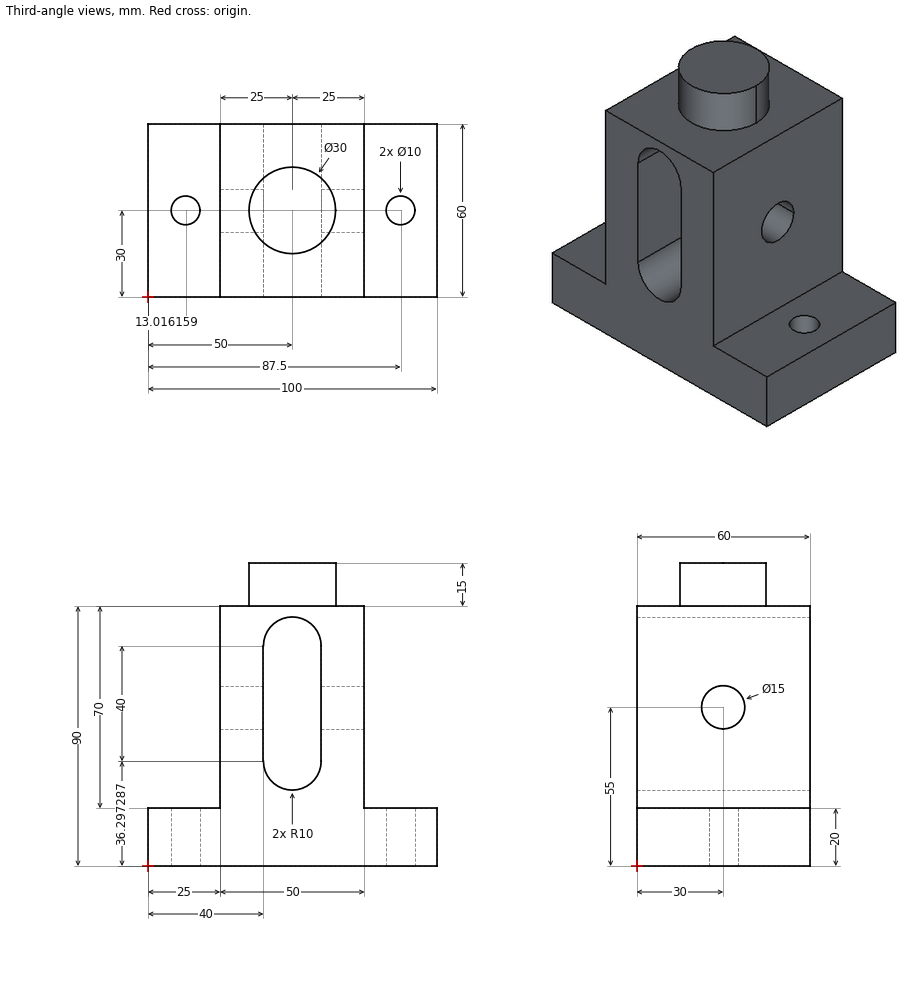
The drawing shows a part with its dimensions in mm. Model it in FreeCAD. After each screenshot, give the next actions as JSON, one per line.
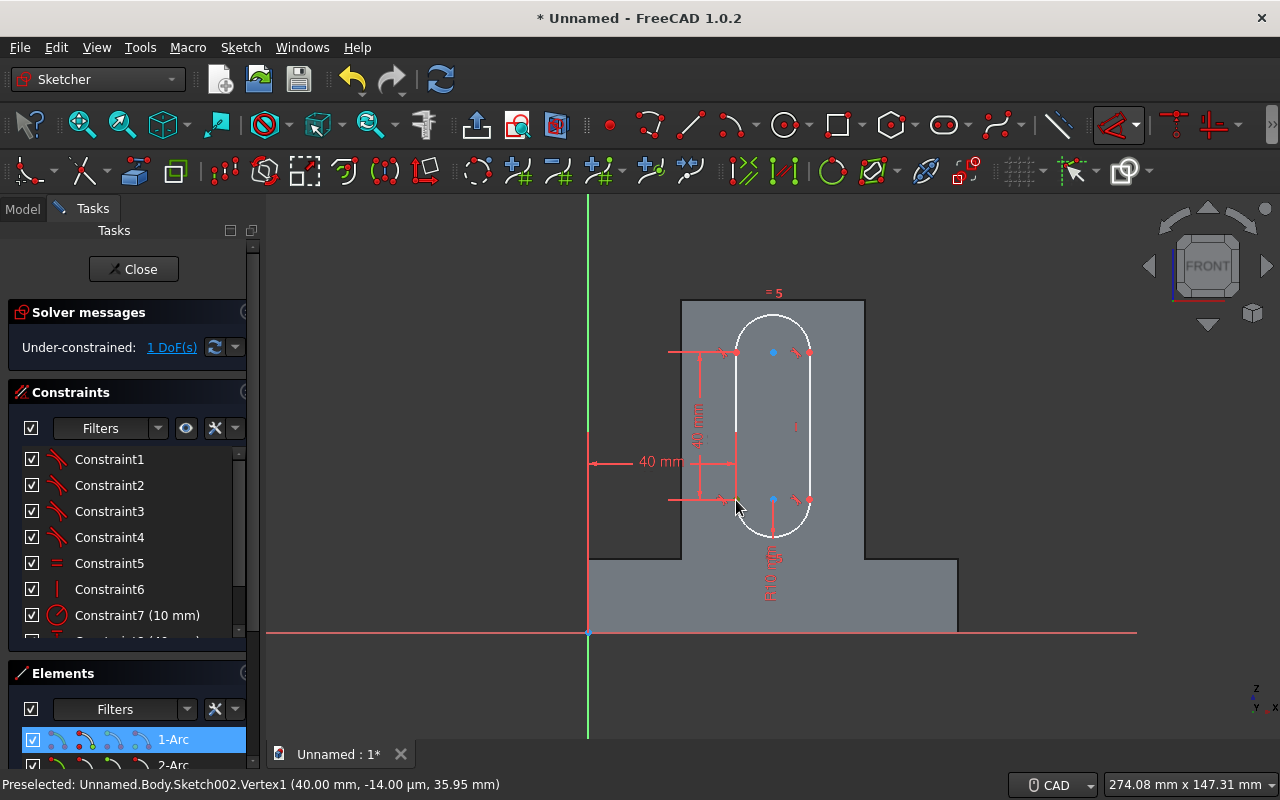
{"action": "left_click", "coordinate": [1138, 126]}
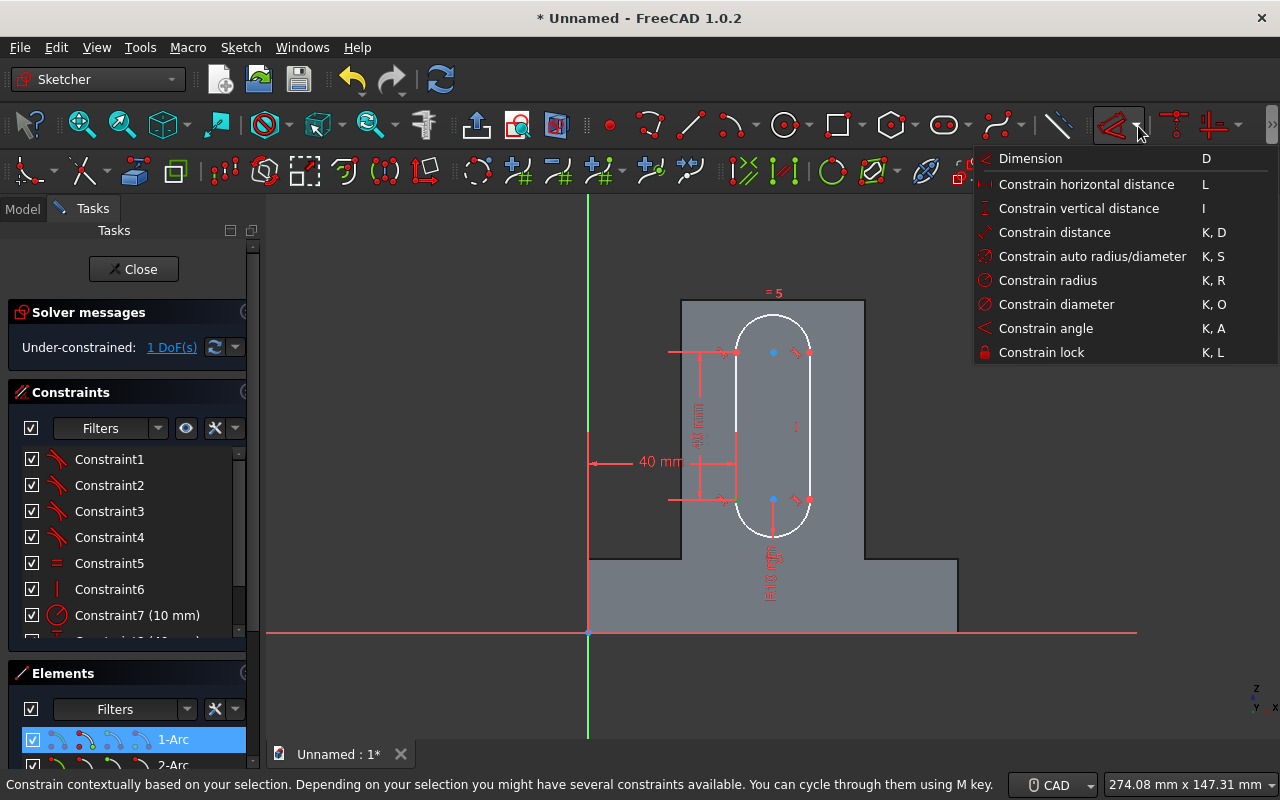
{"action": "left_click", "coordinate": [1126, 208]}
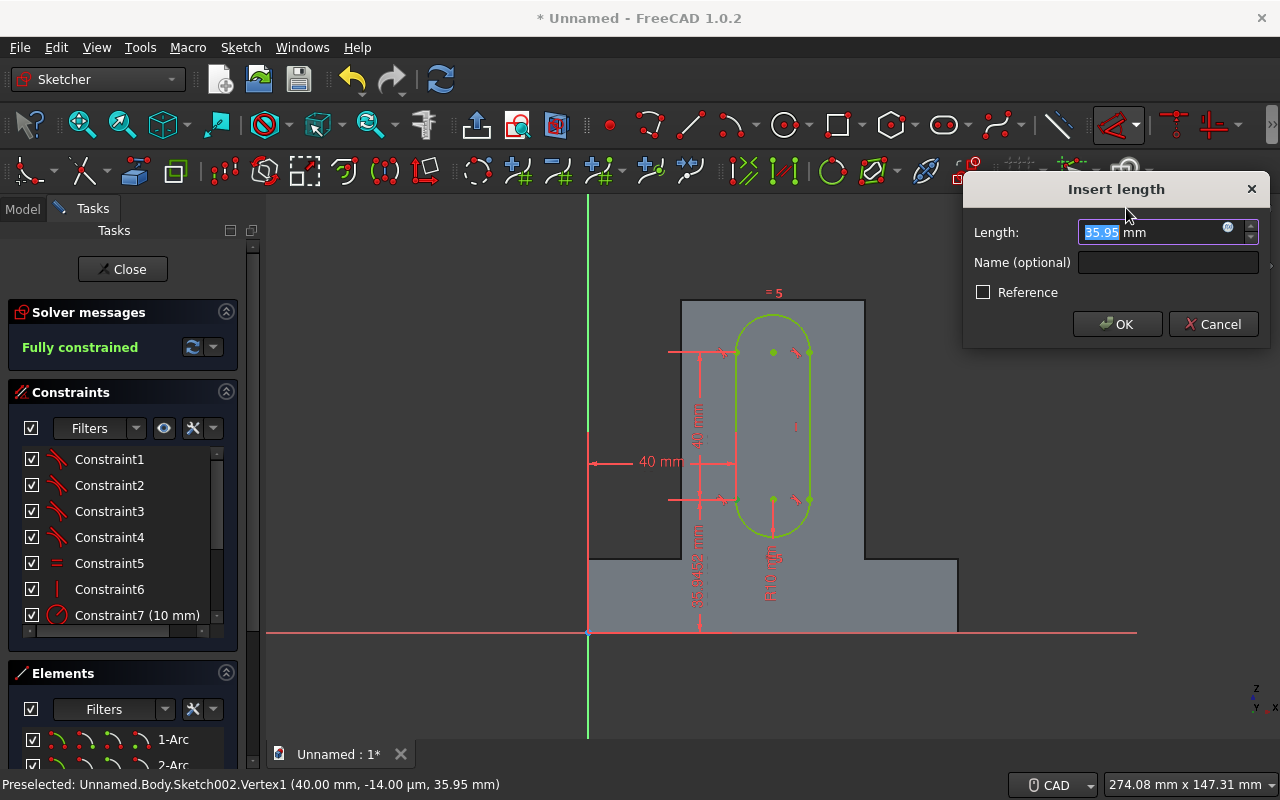
{"action": "type", "text": "36.297287"}
{"action": "key", "text": "Return"}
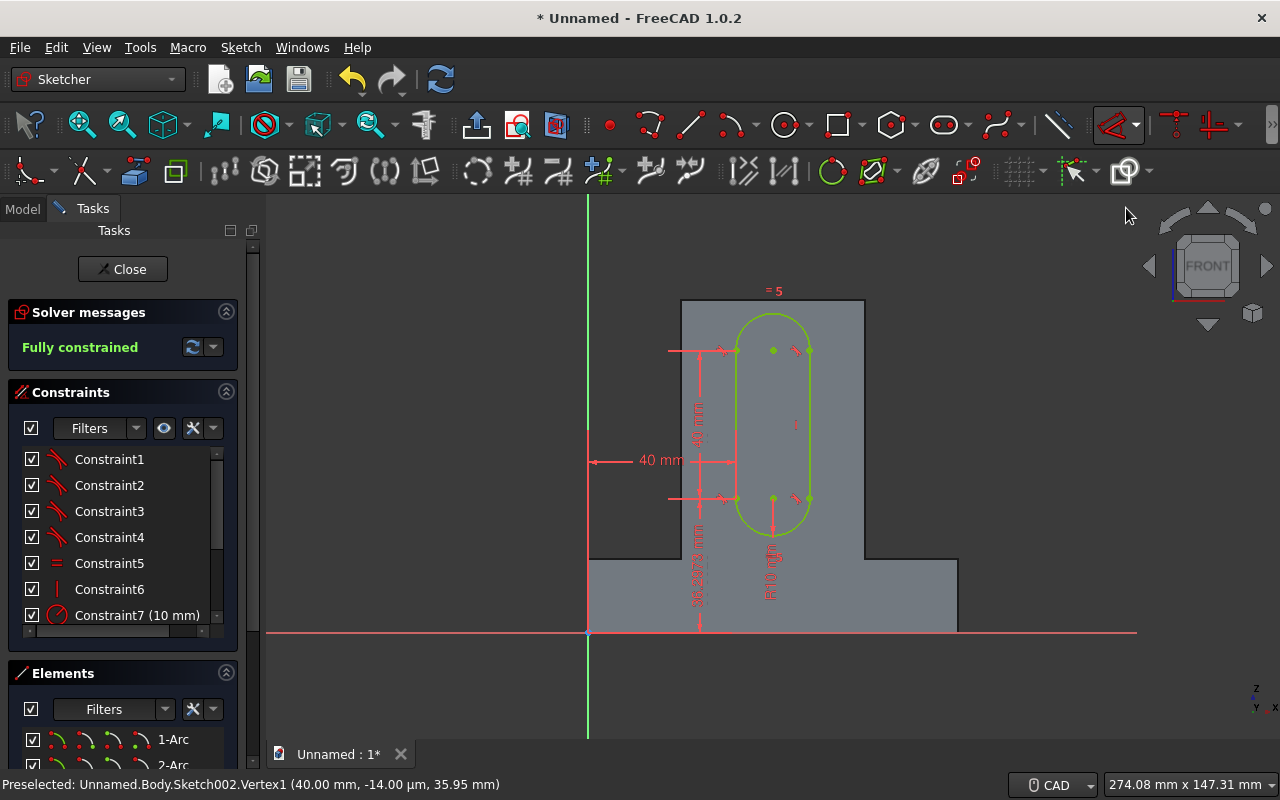
{"action": "left_click", "coordinate": [123, 269]}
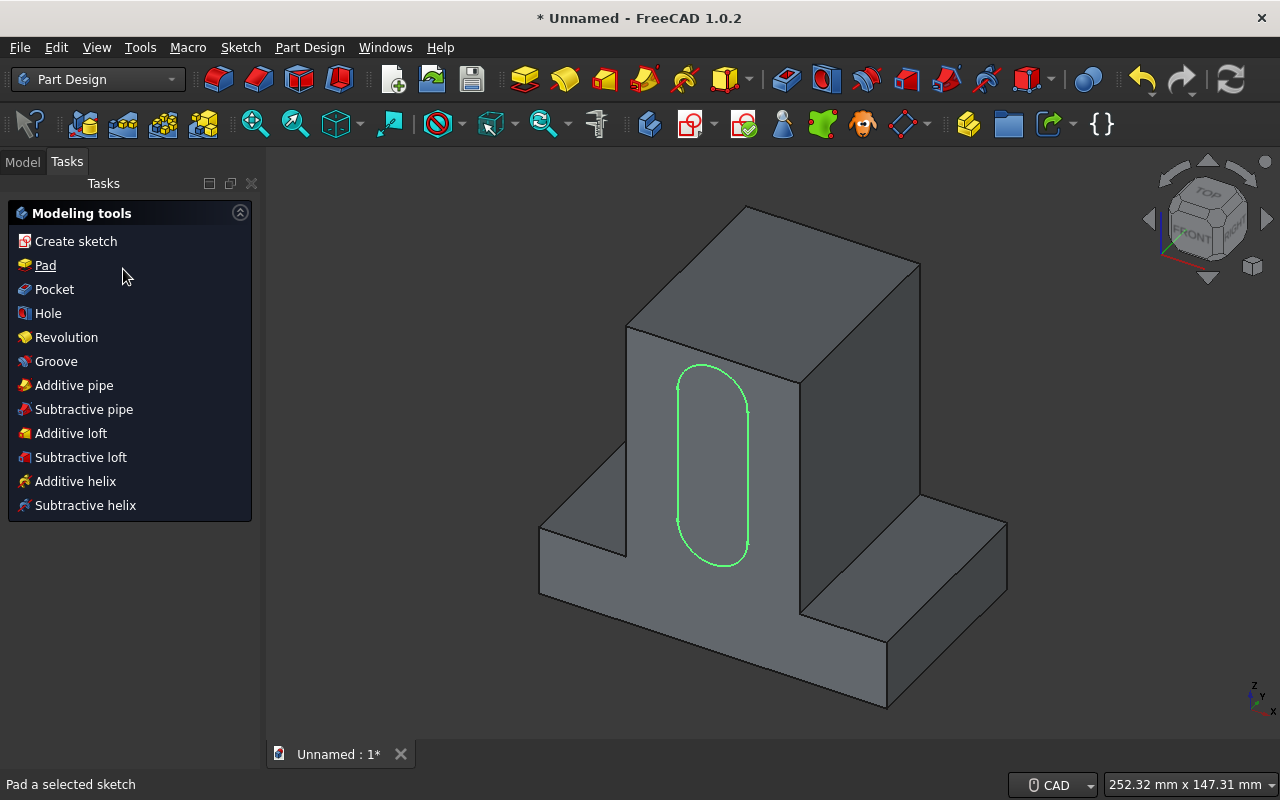
{"action": "left_click", "coordinate": [788, 80]}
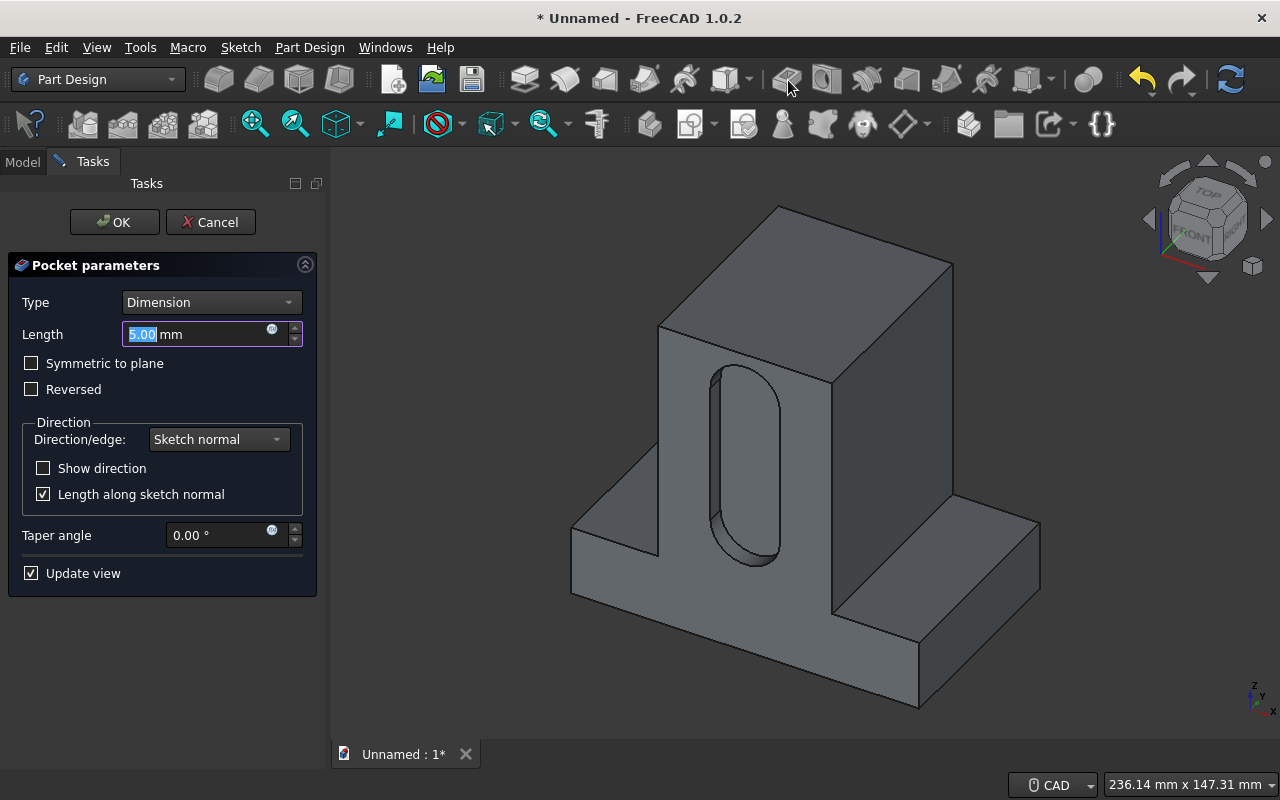
{"action": "type", "text": "60"}
{"action": "key", "text": "Tab"}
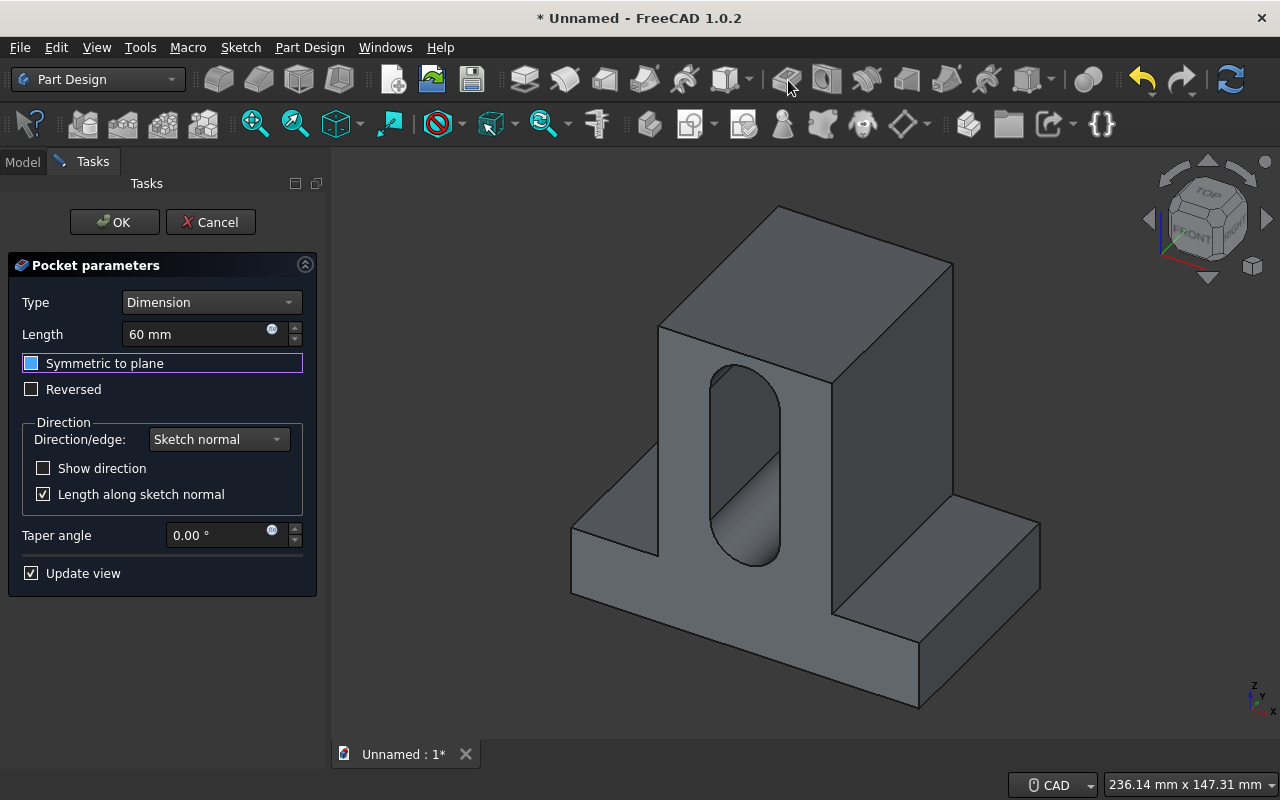
{"action": "left_click", "coordinate": [115, 222]}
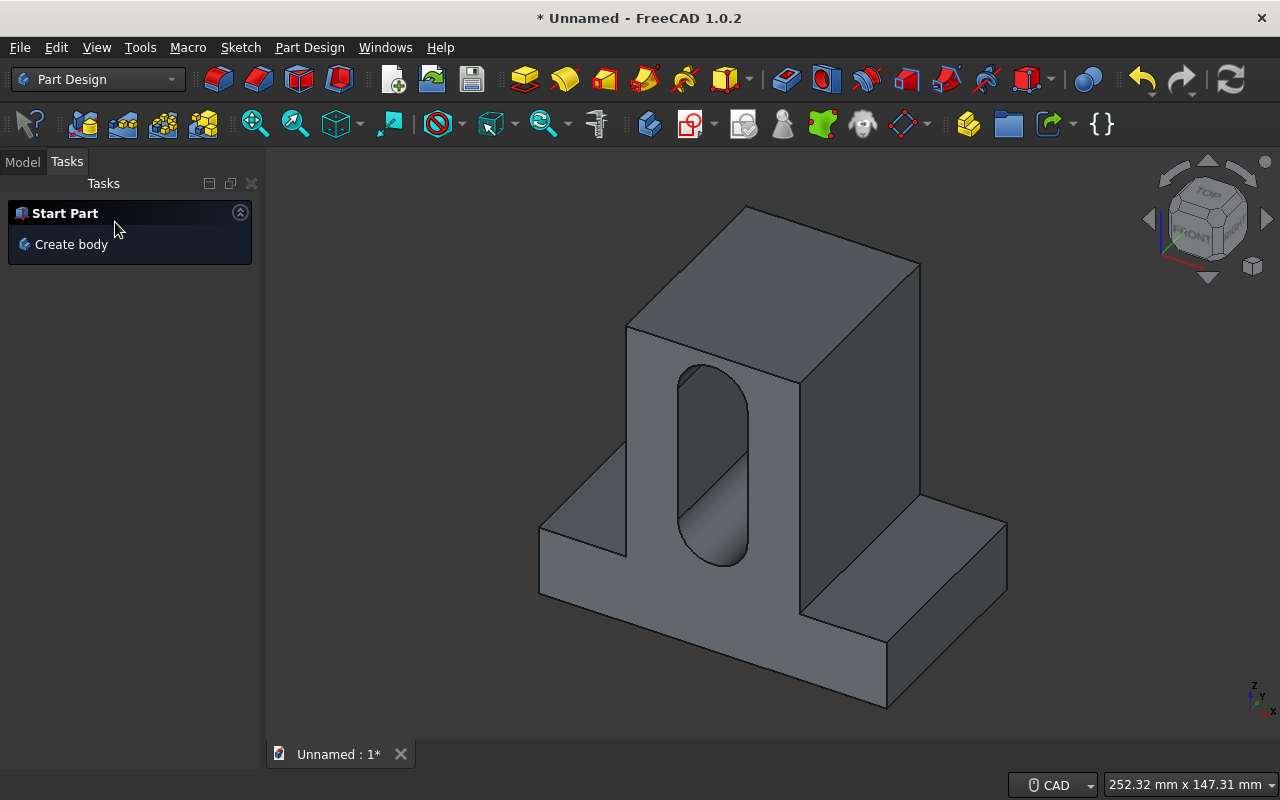
{"action": "left_click", "coordinate": [608, 515]}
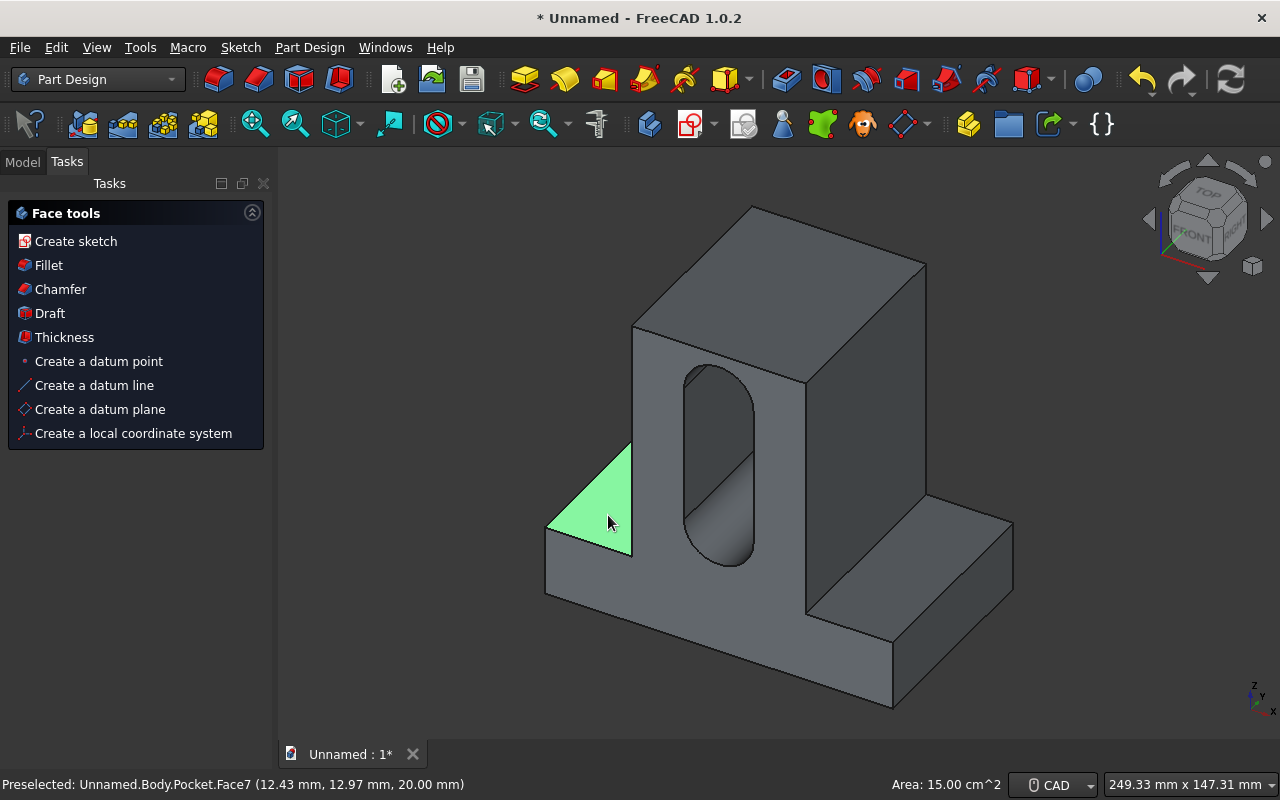
{"action": "left_click", "coordinate": [690, 124]}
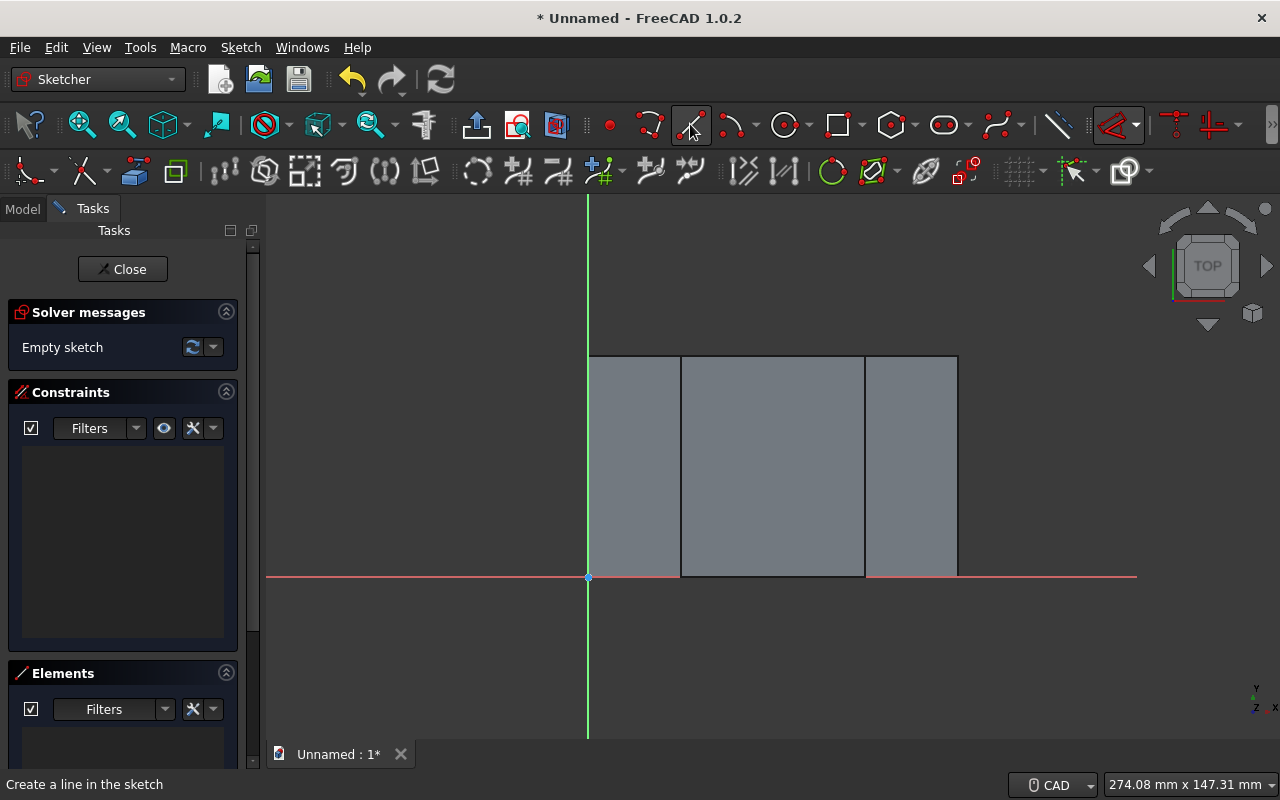
{"action": "scroll", "coordinate": [826, 569], "scroll_direction": "up", "scroll_amount": 3}